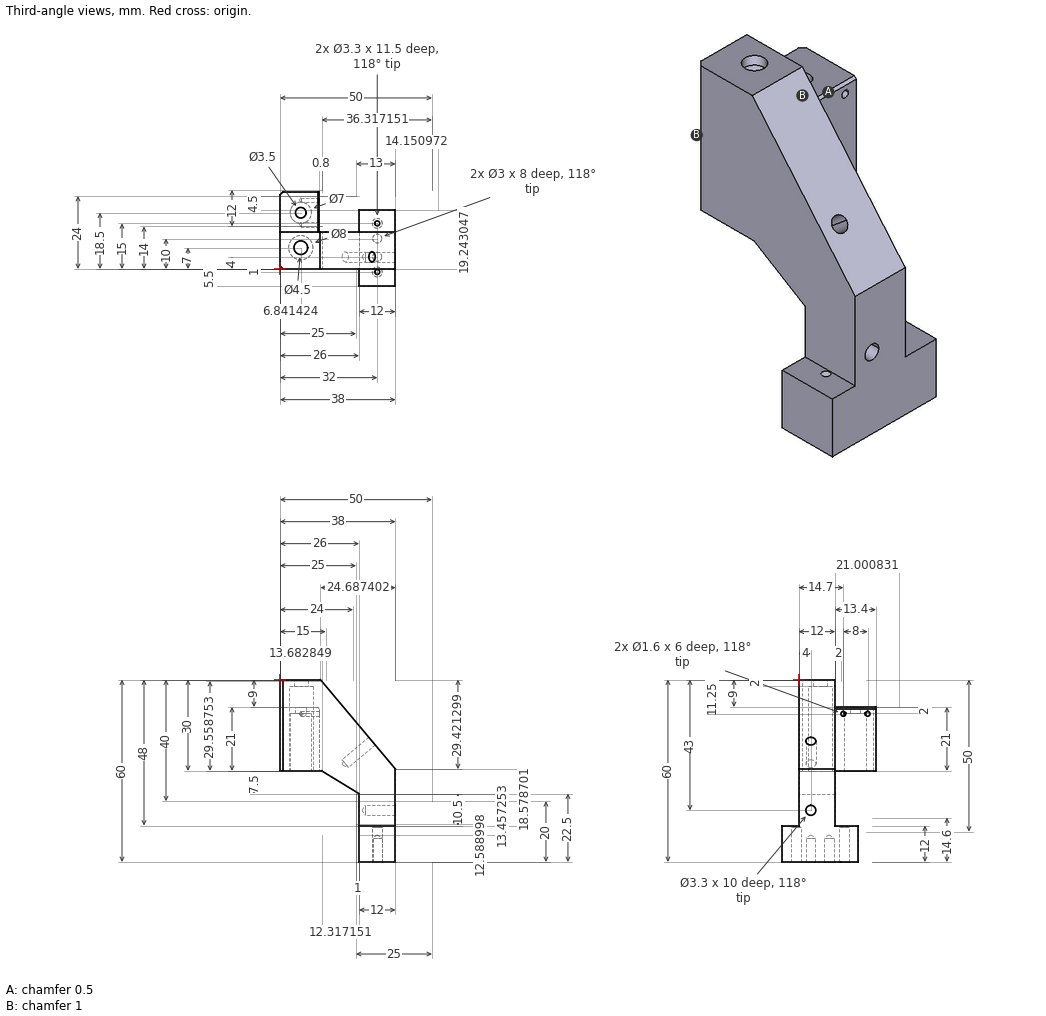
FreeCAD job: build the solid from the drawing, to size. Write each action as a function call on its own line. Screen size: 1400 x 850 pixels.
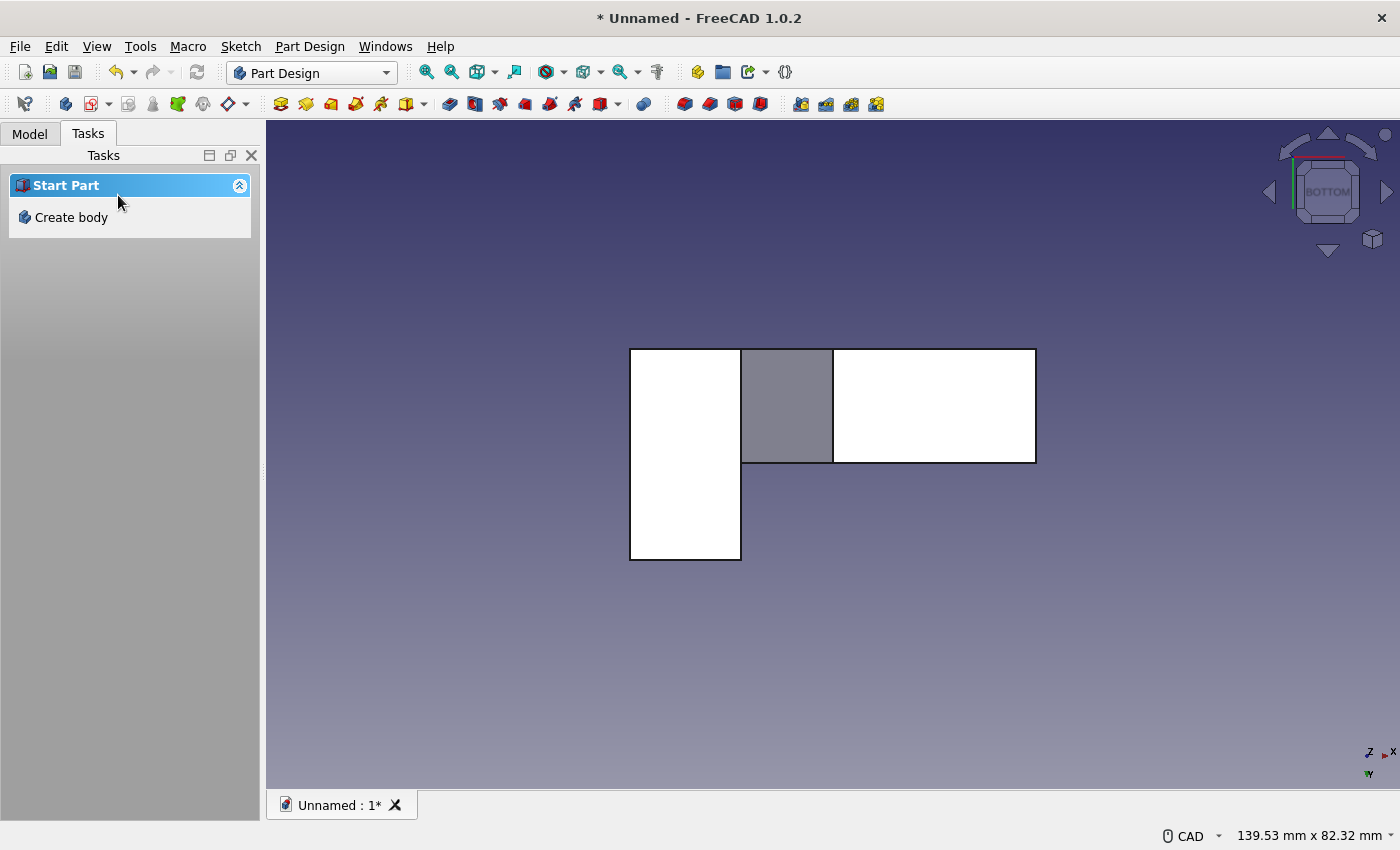
click(427, 72)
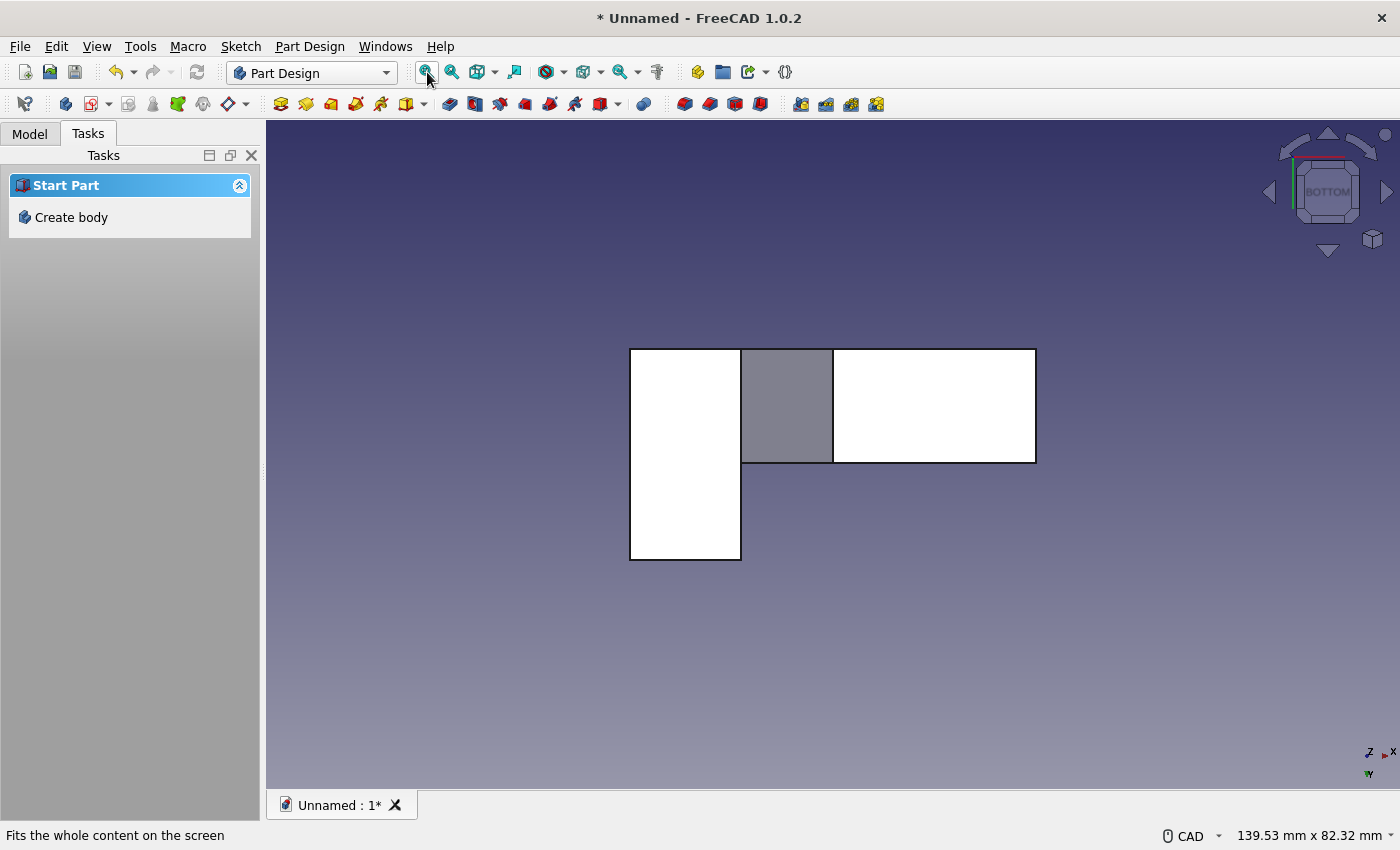
click(90, 104)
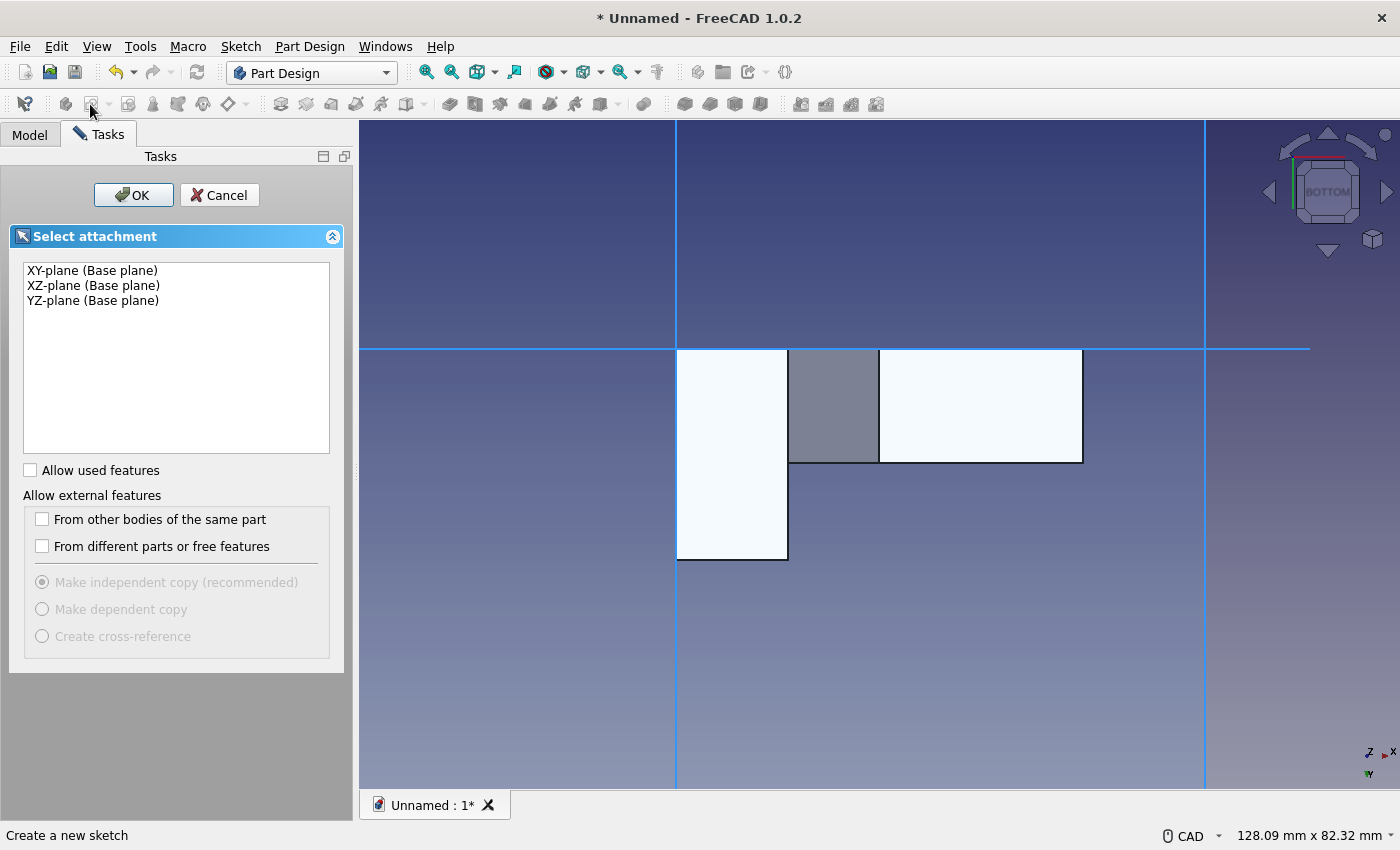
click(84, 270)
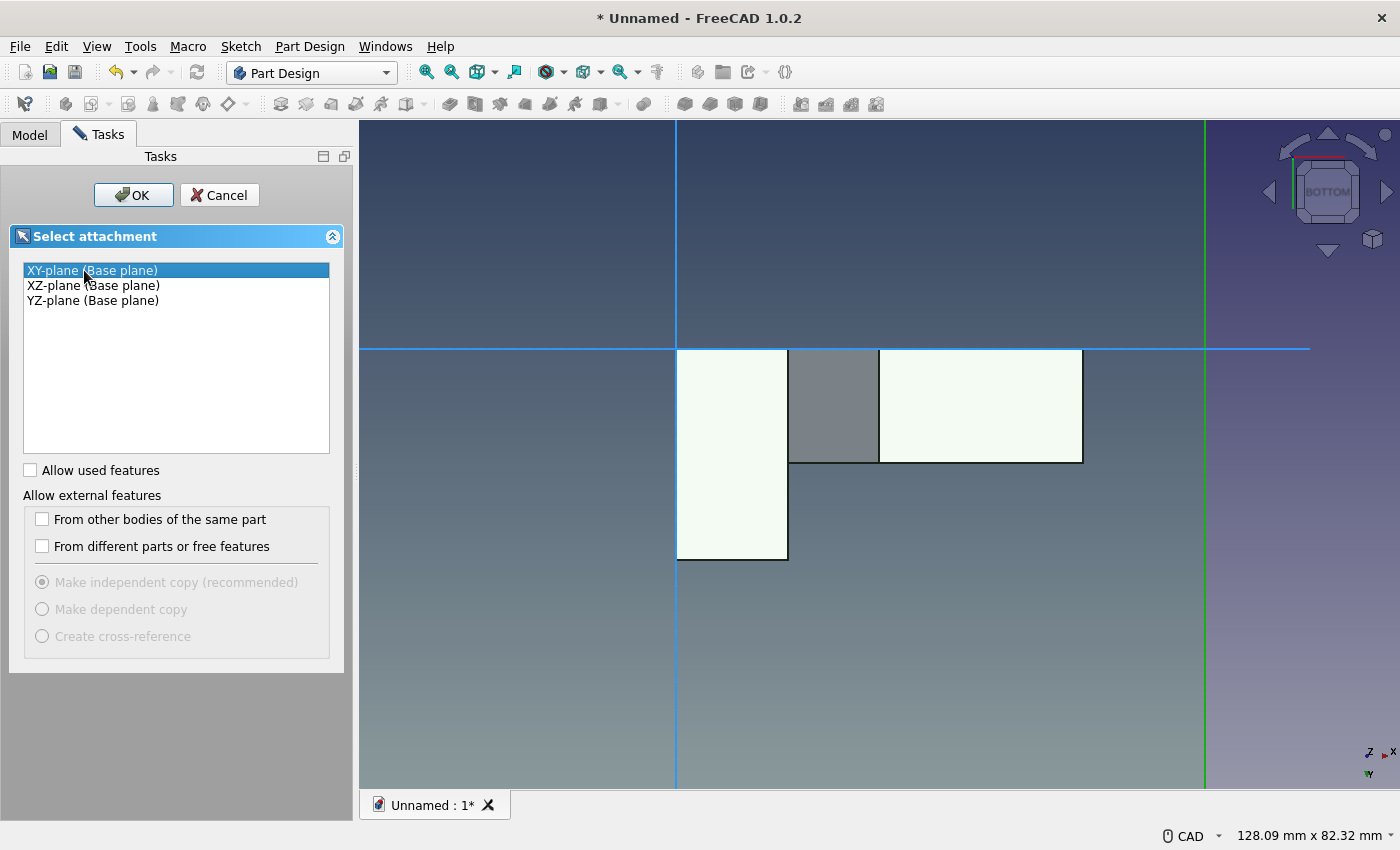
click(134, 195)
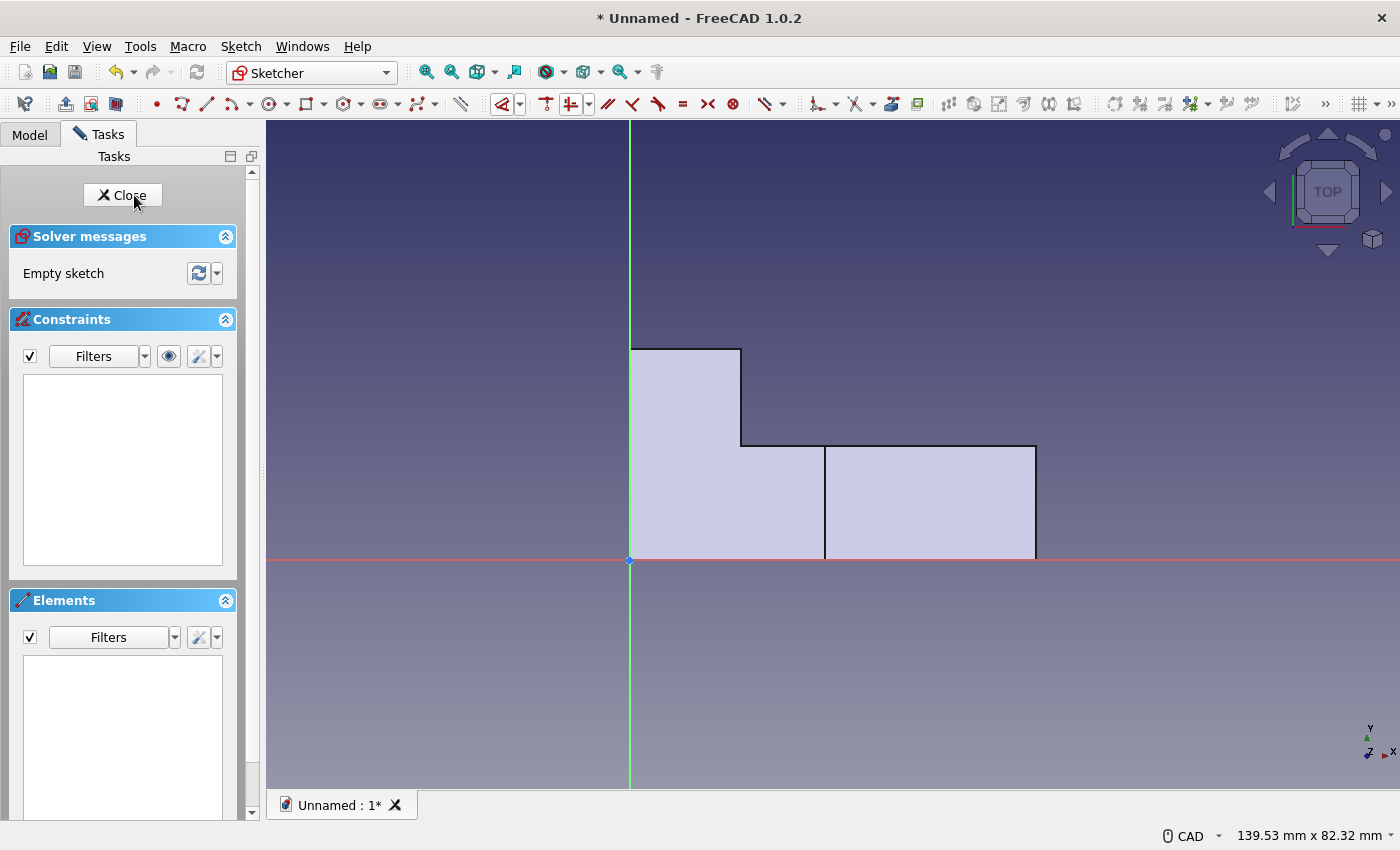
scroll(600, 484, up, 4)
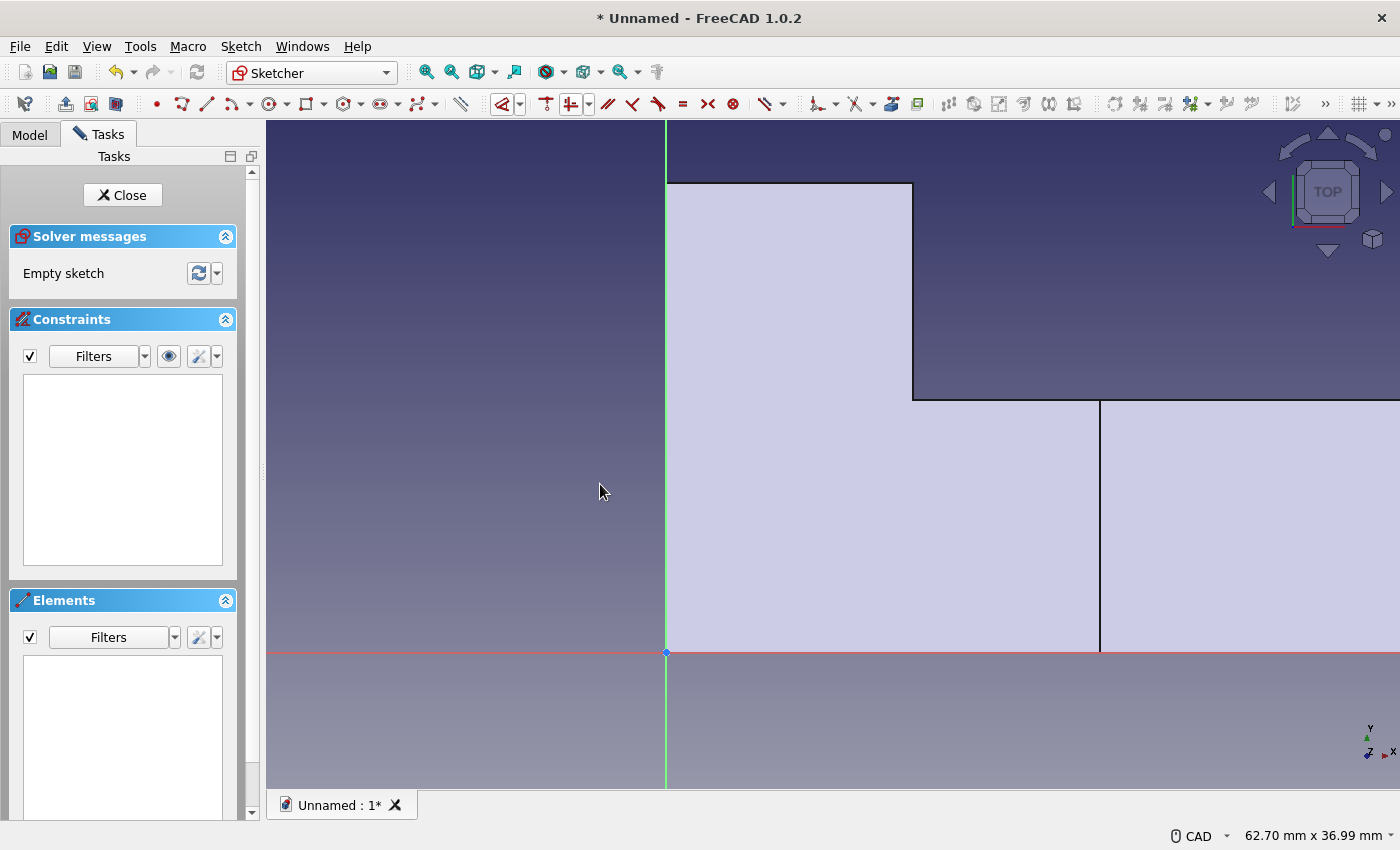
click(268, 104)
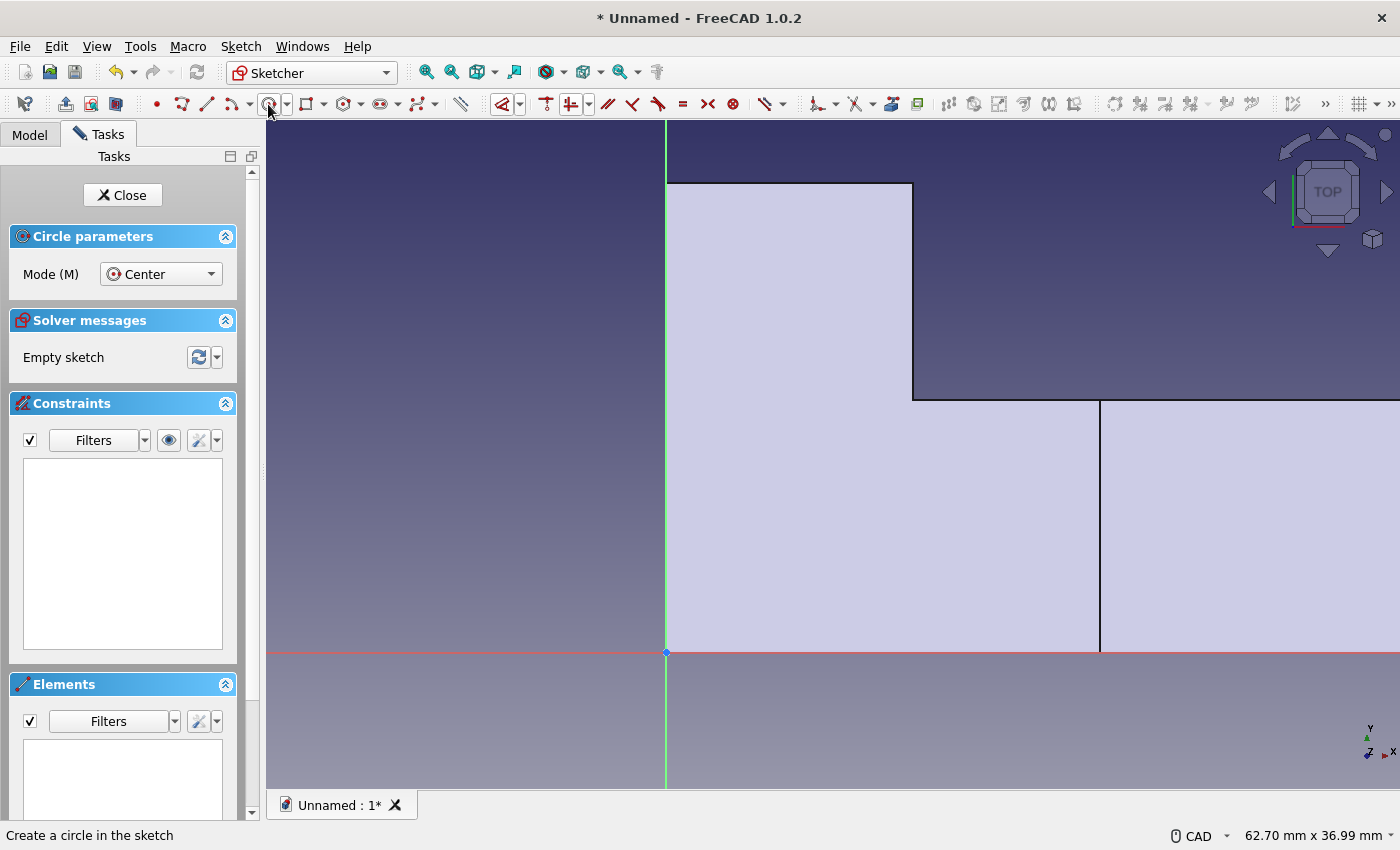
click(790, 526)
click(841, 475)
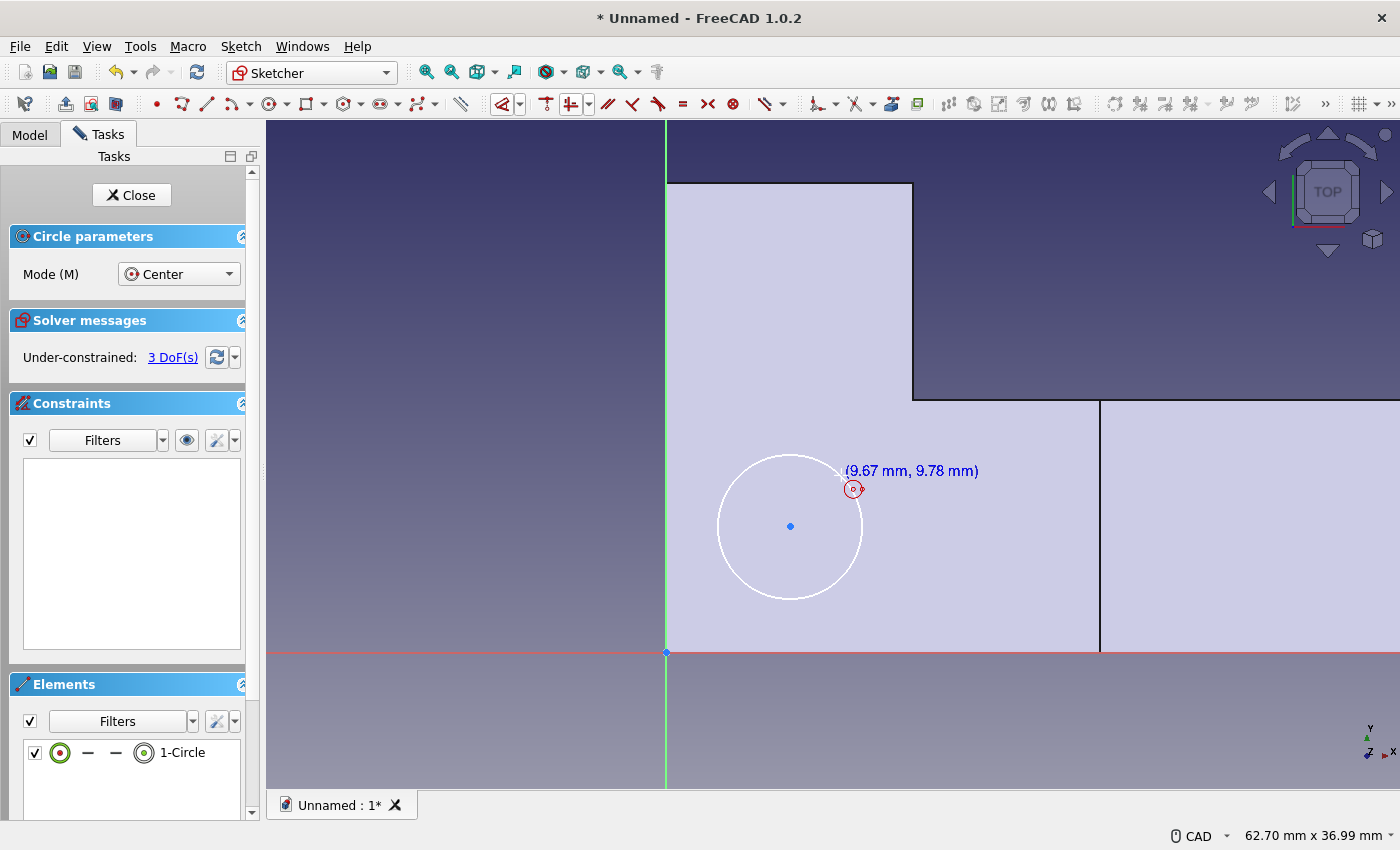
click(790, 318)
click(835, 273)
key(Escape)